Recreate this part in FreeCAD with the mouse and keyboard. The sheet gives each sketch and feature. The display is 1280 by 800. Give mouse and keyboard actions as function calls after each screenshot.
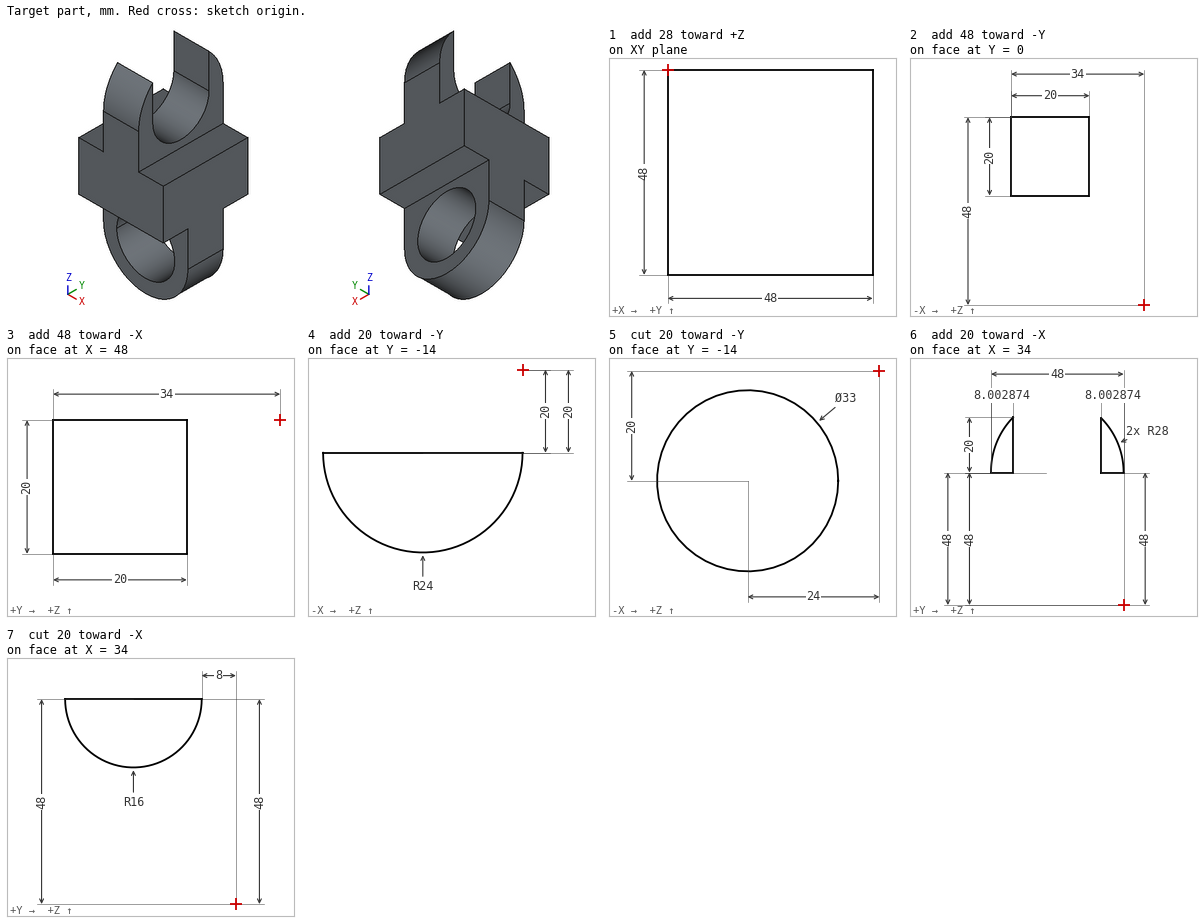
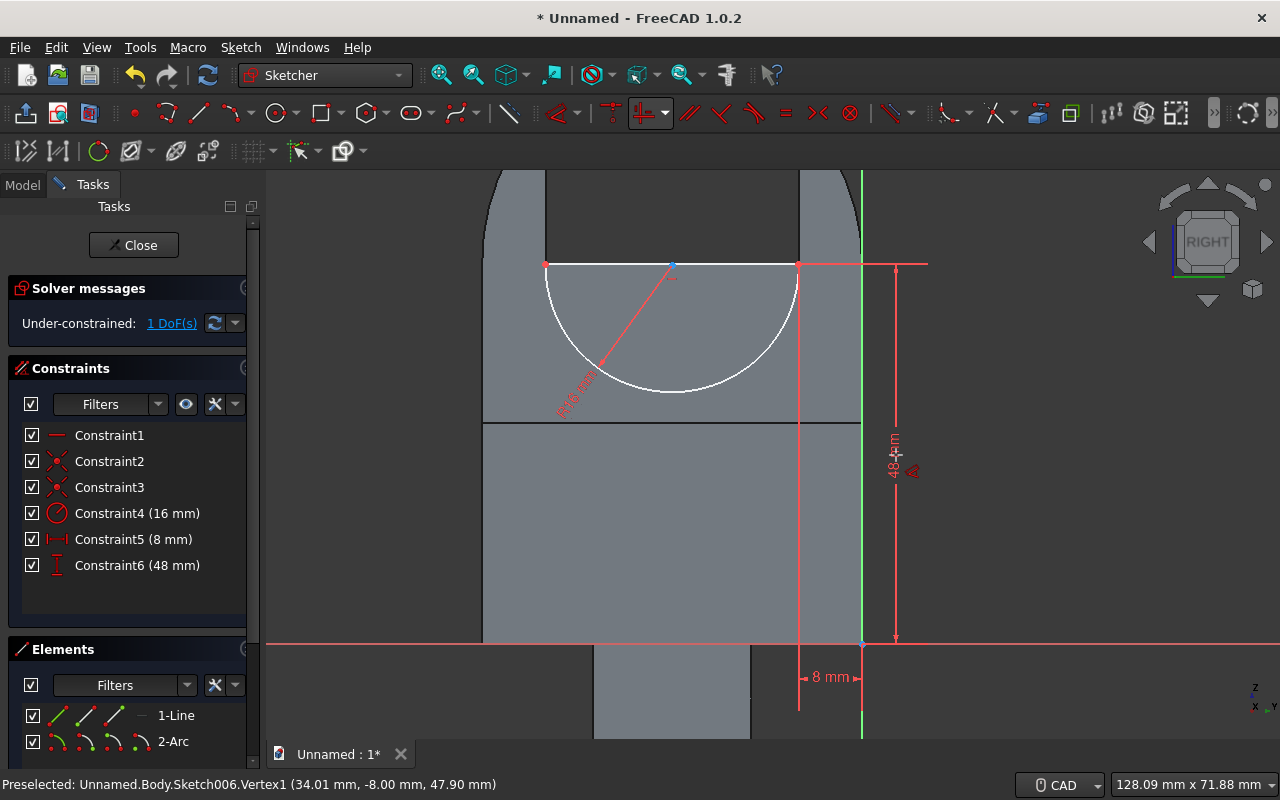
click(672, 265)
click(896, 368)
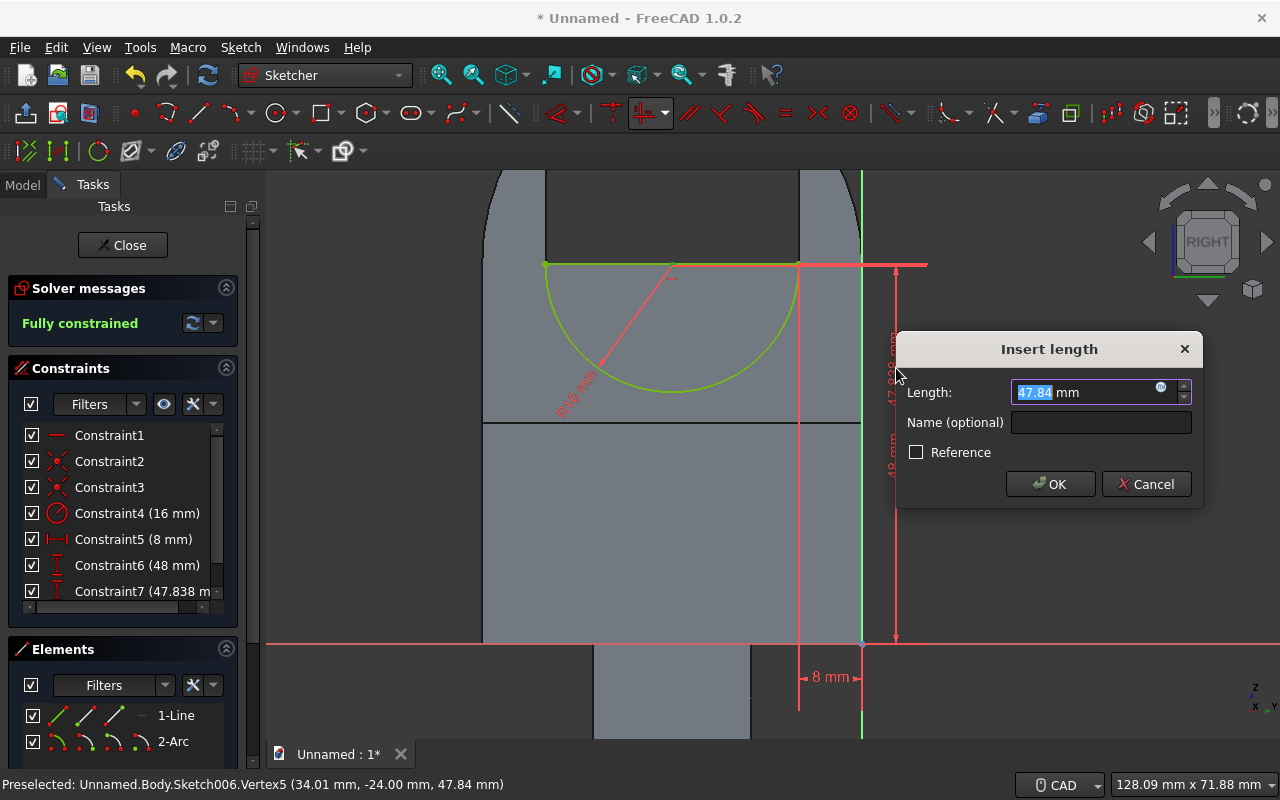
text(48)
key(Return)
key(Escape)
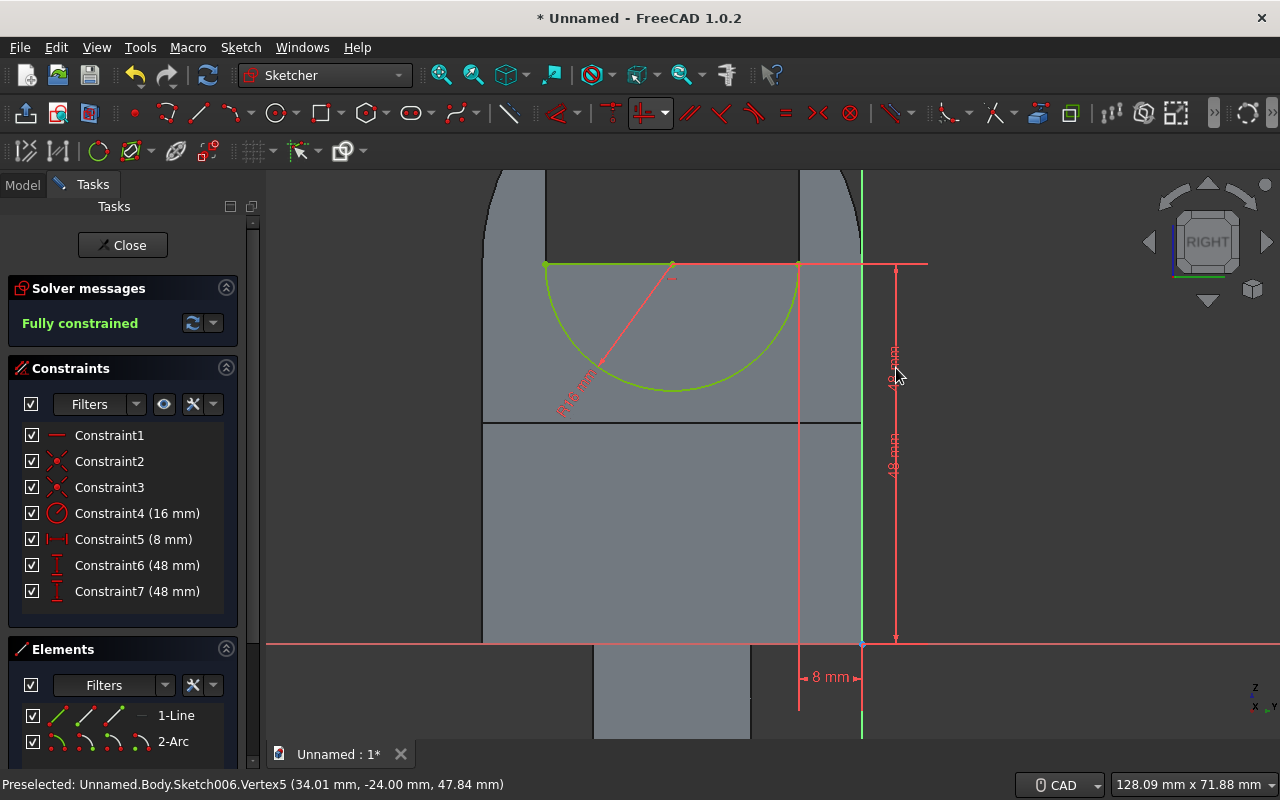
click(123, 245)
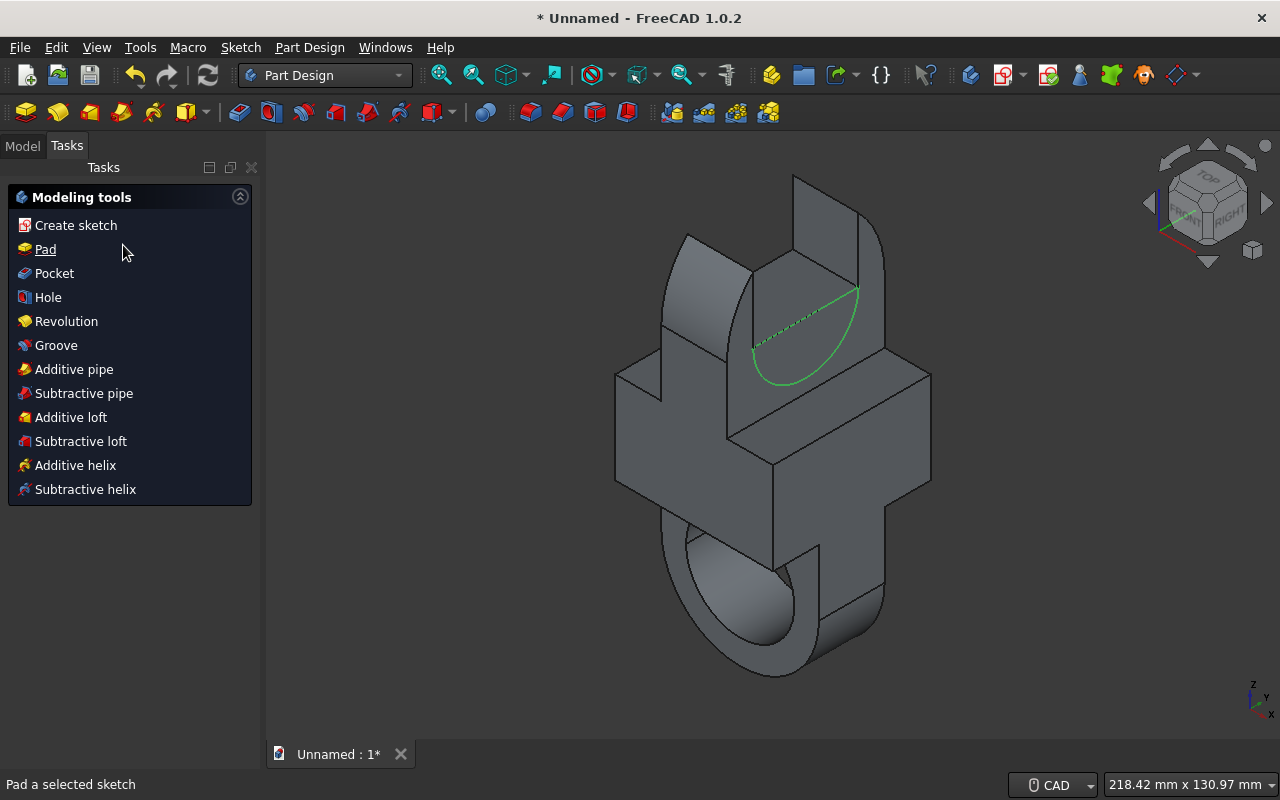
click(240, 112)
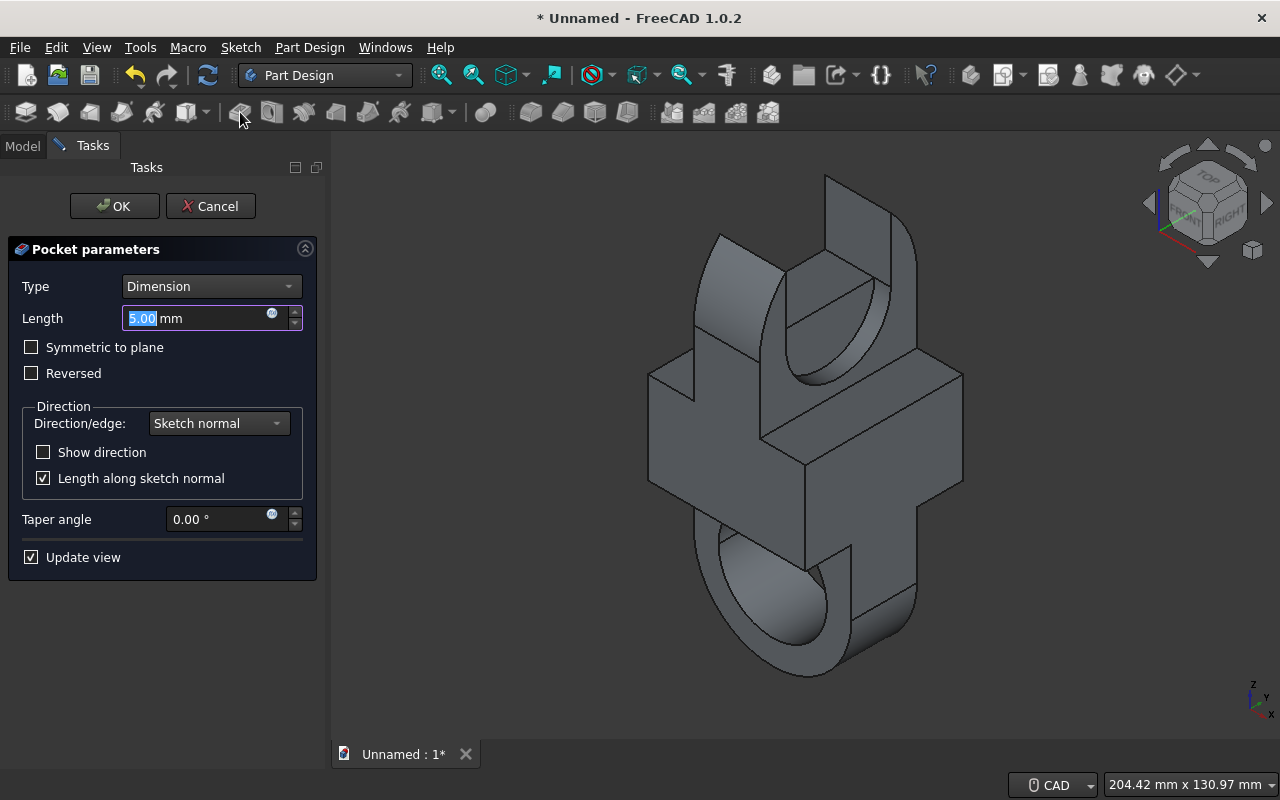
text(20)
key(Tab)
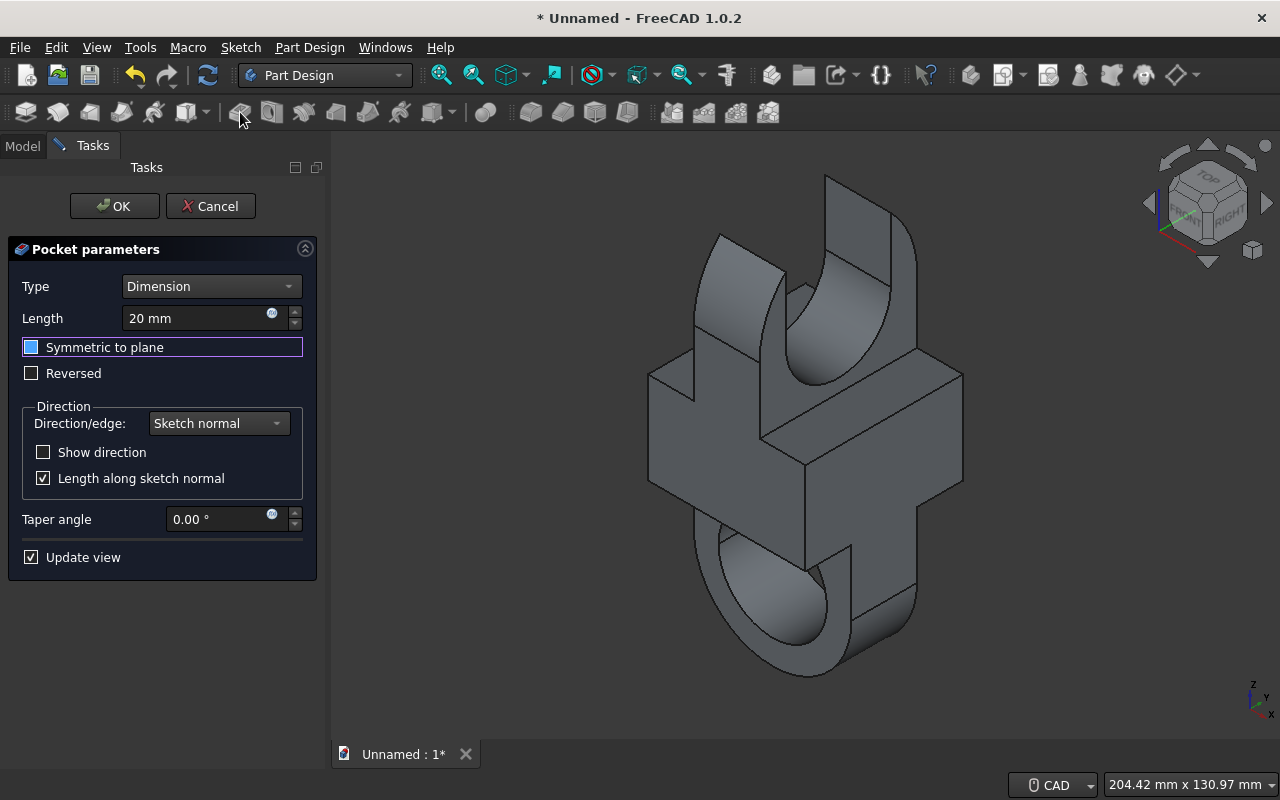
click(115, 206)